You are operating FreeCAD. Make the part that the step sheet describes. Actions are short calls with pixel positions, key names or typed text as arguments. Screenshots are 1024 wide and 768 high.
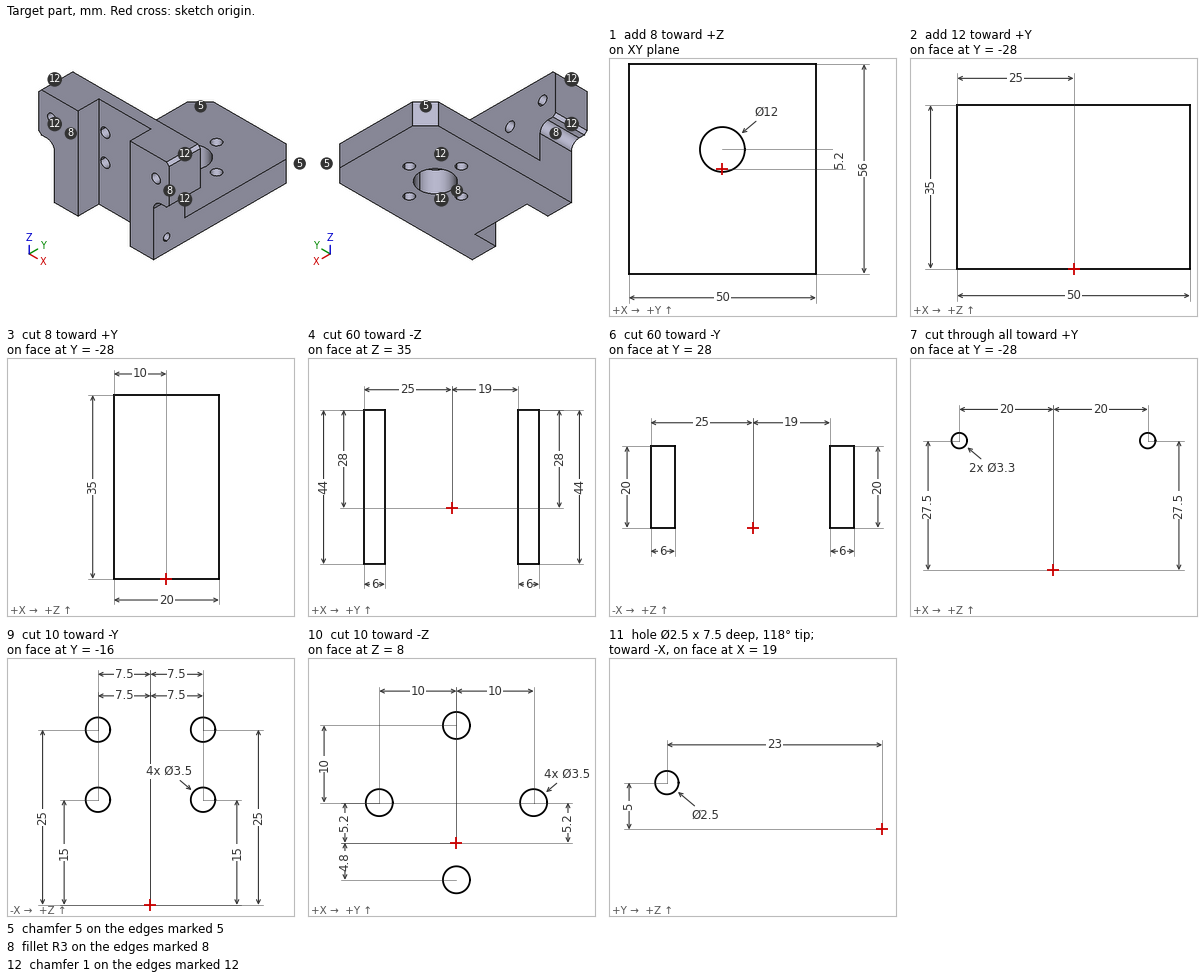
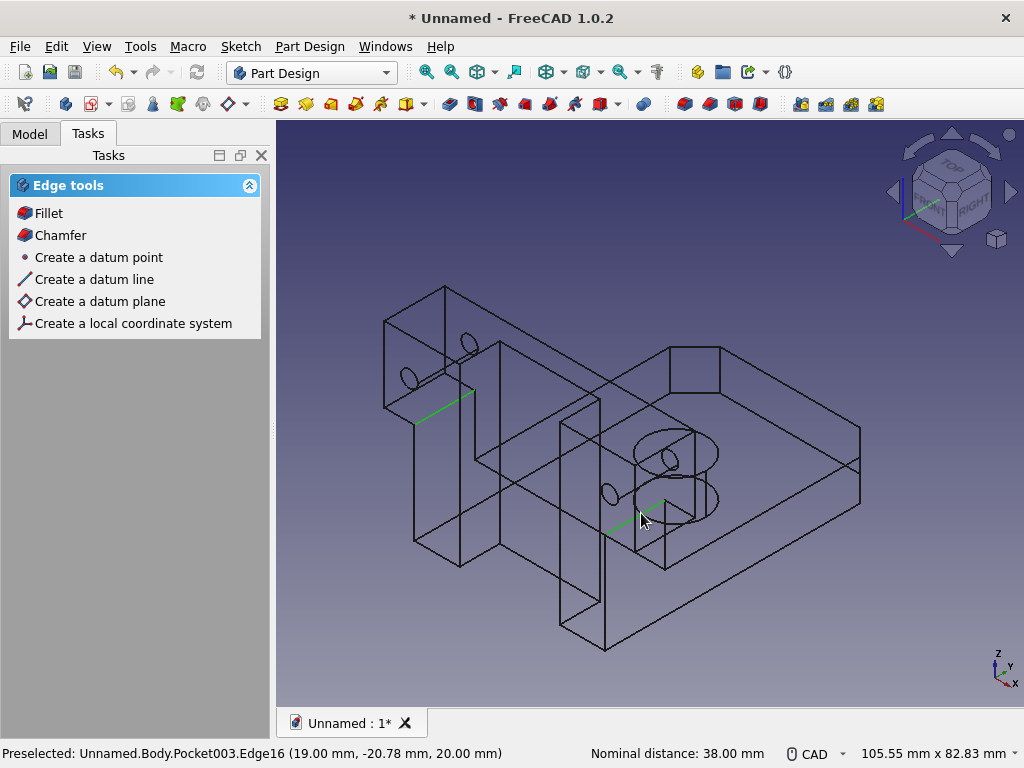
key(v)
key(1)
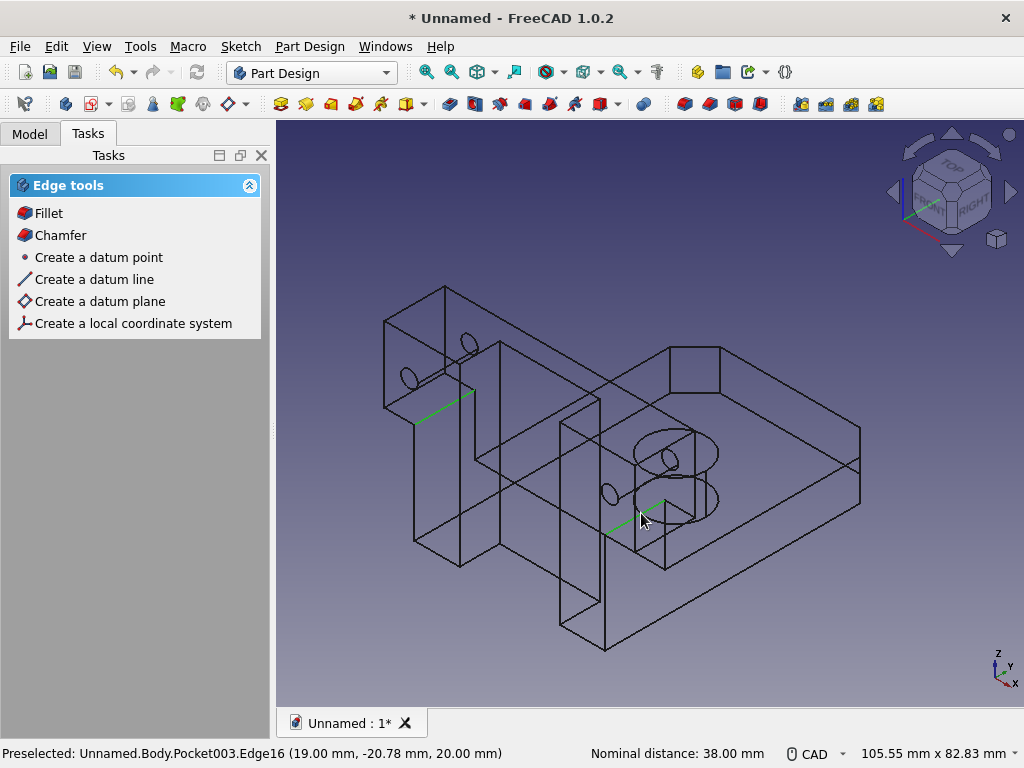
click(685, 104)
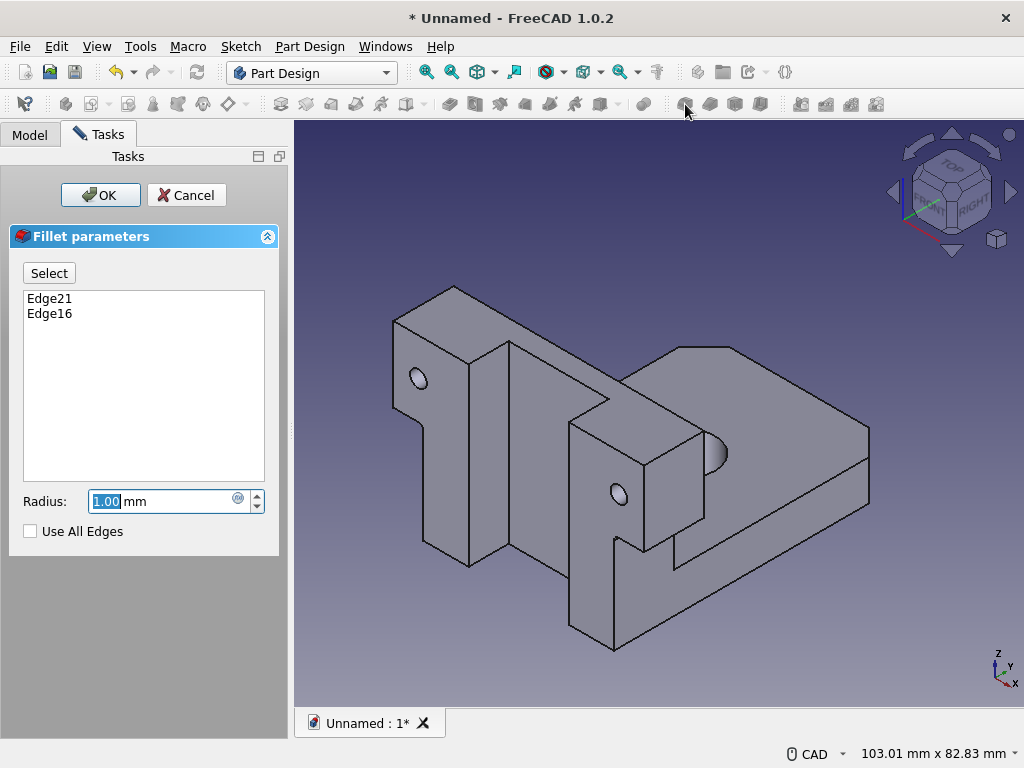
text(3)
key(Tab)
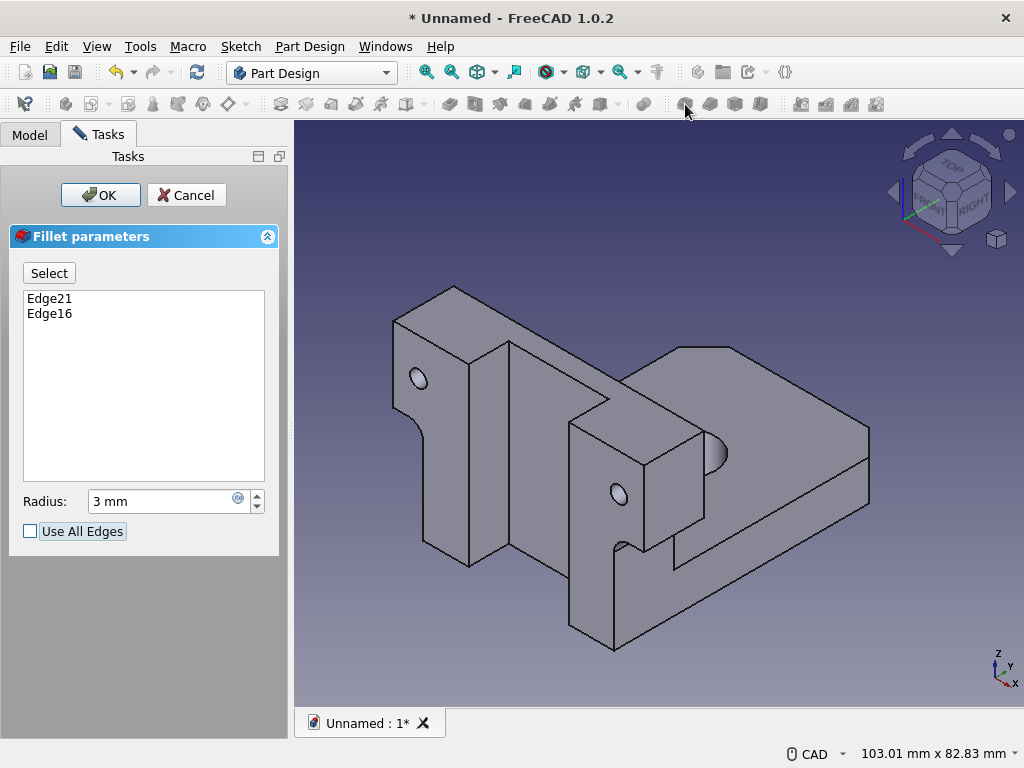
click(101, 195)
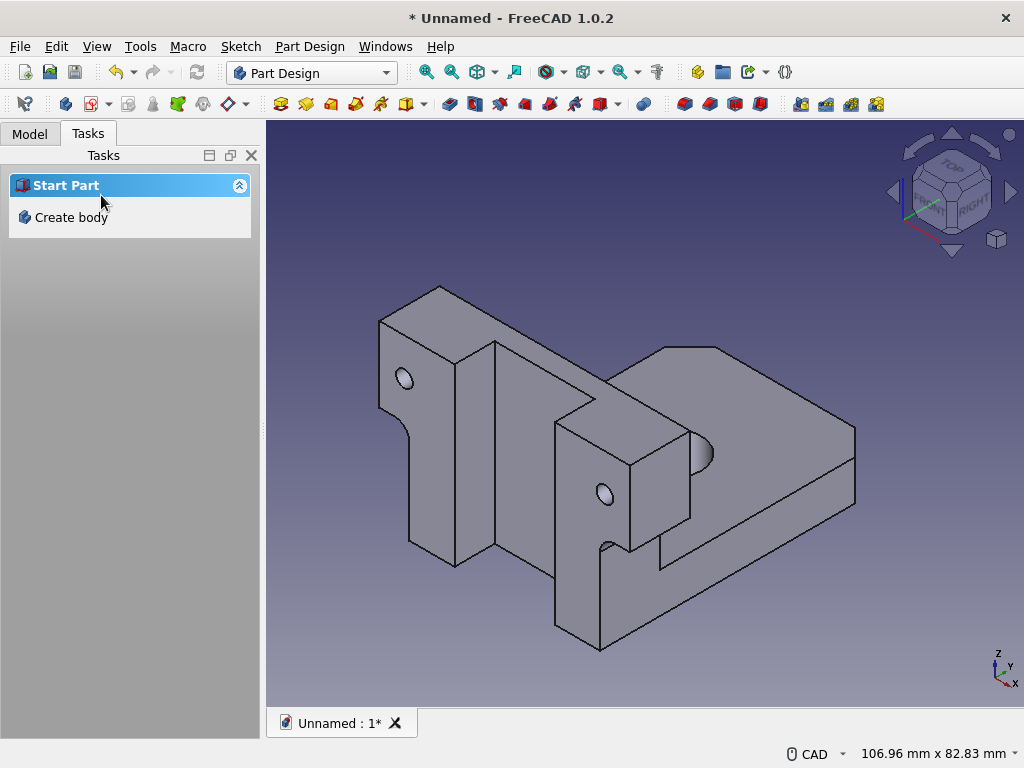
key(4)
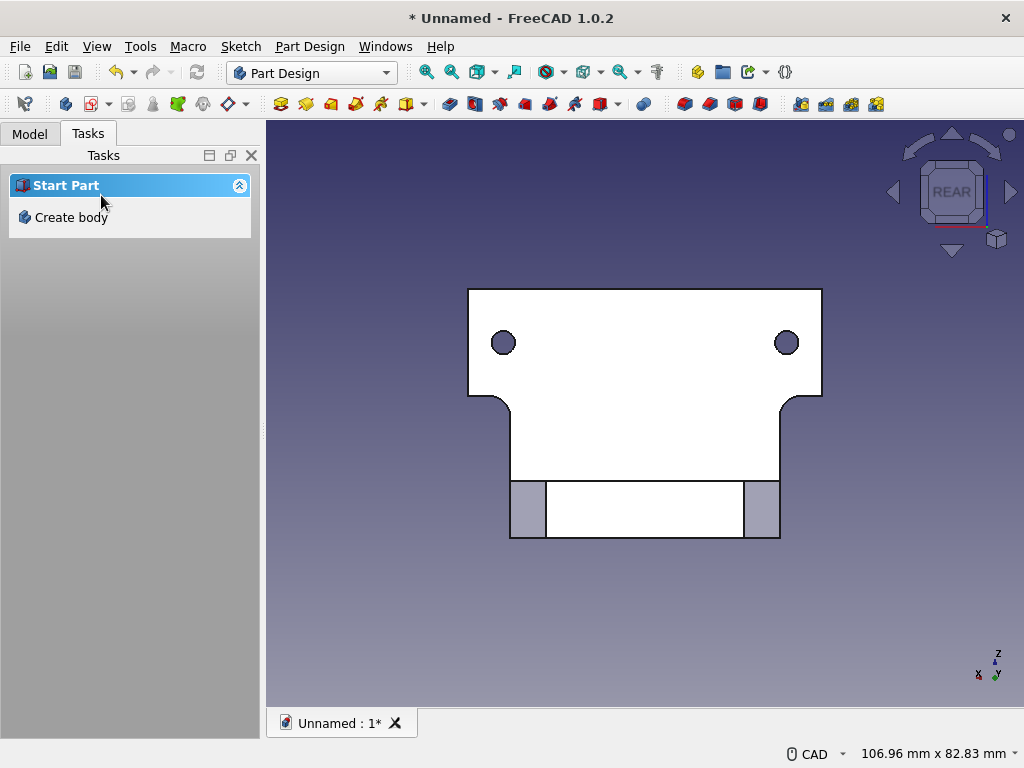
click(645, 384)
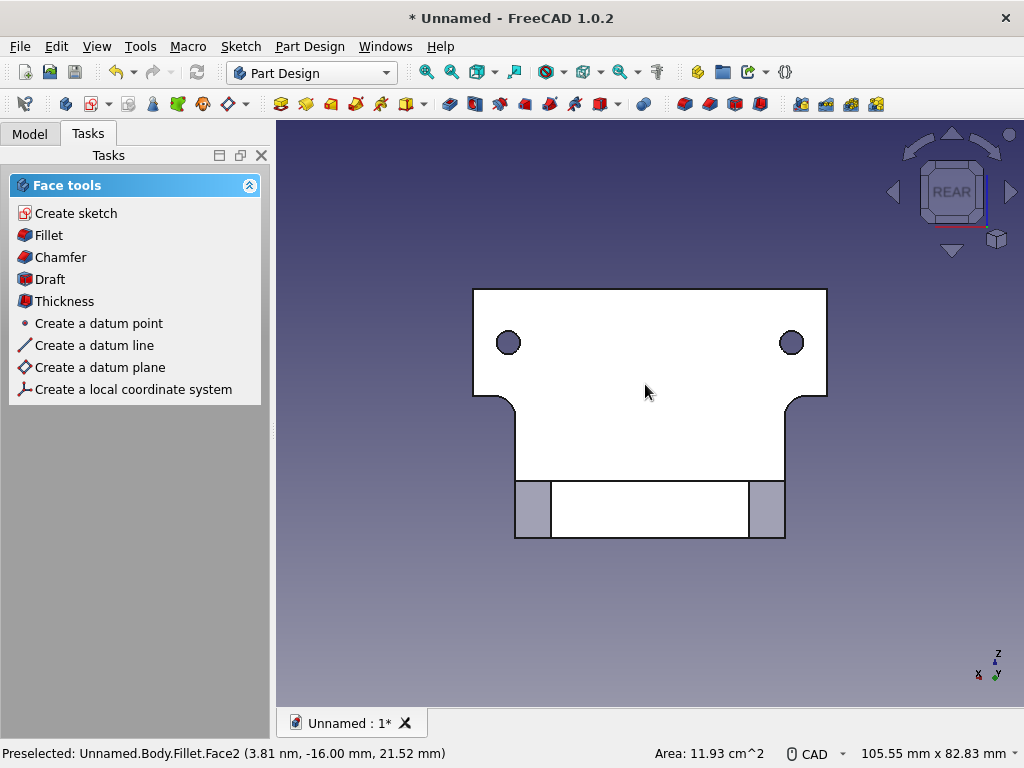
click(90, 104)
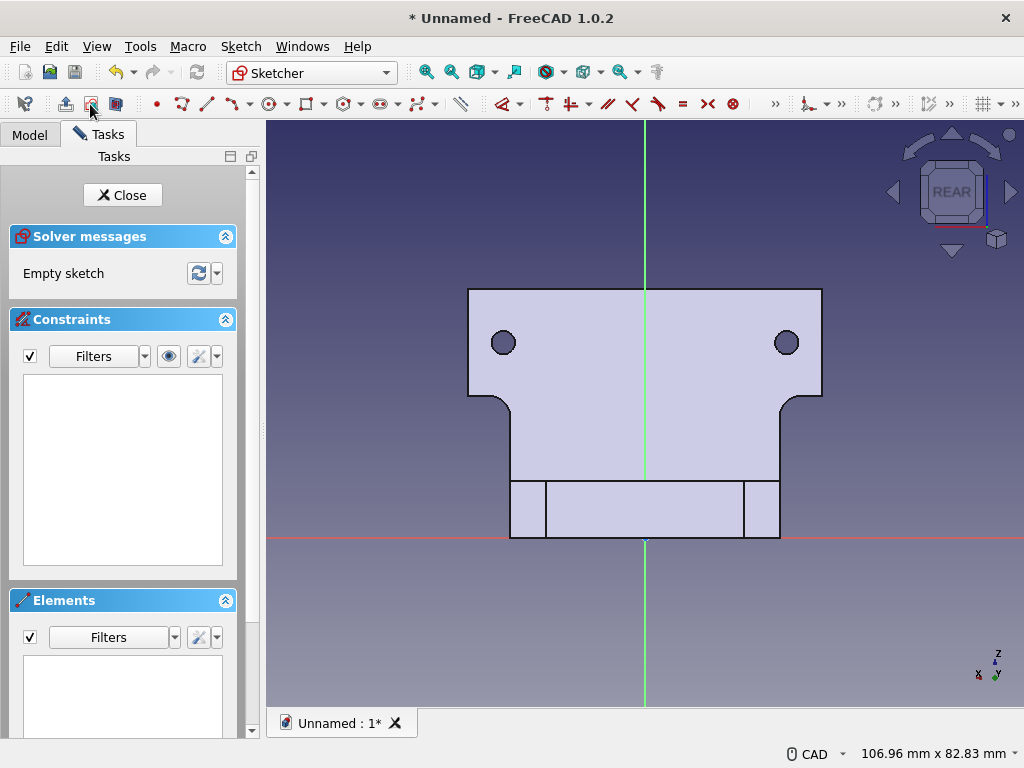
click(116, 104)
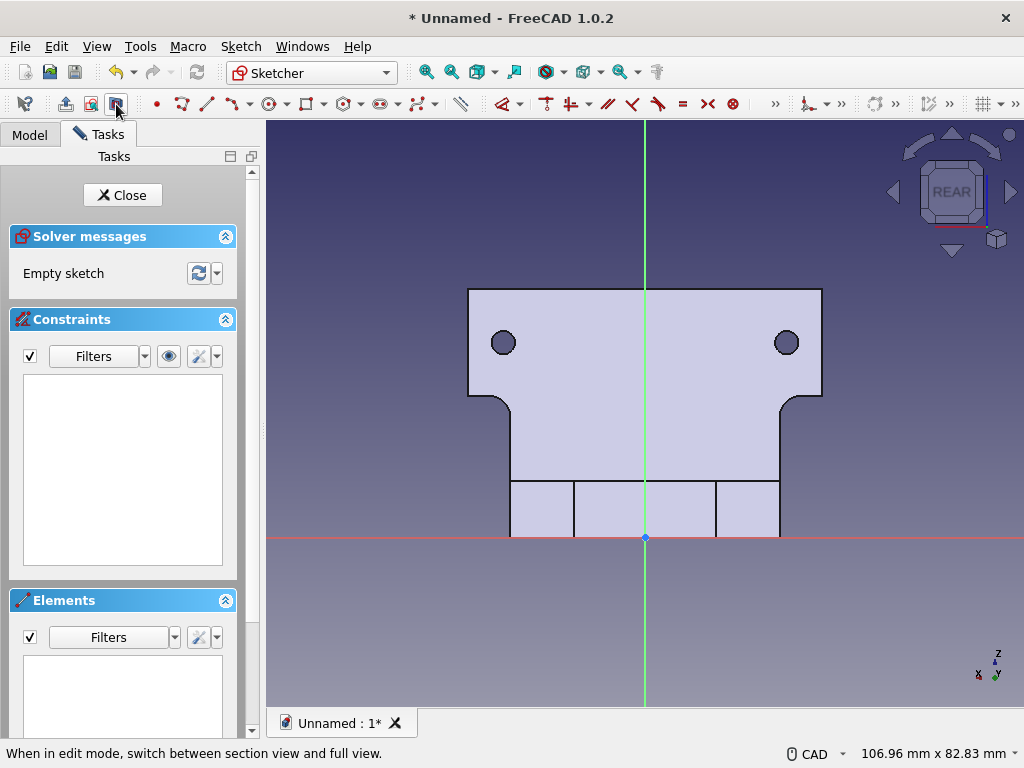
scroll(728, 478, up, 3)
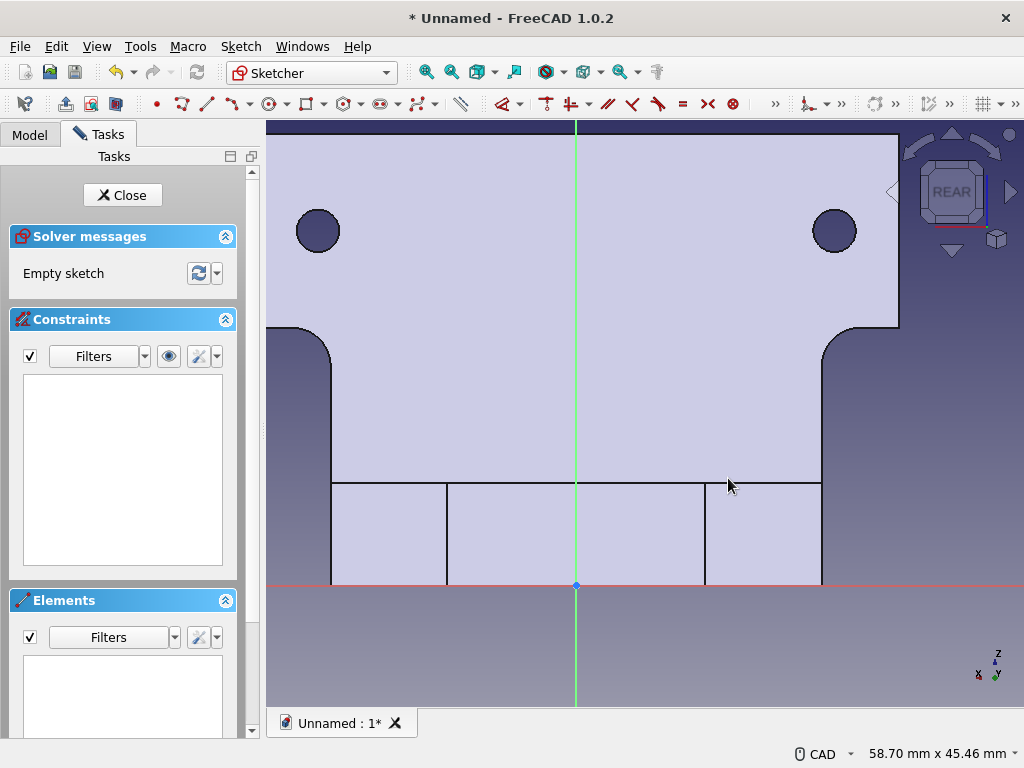
click(268, 104)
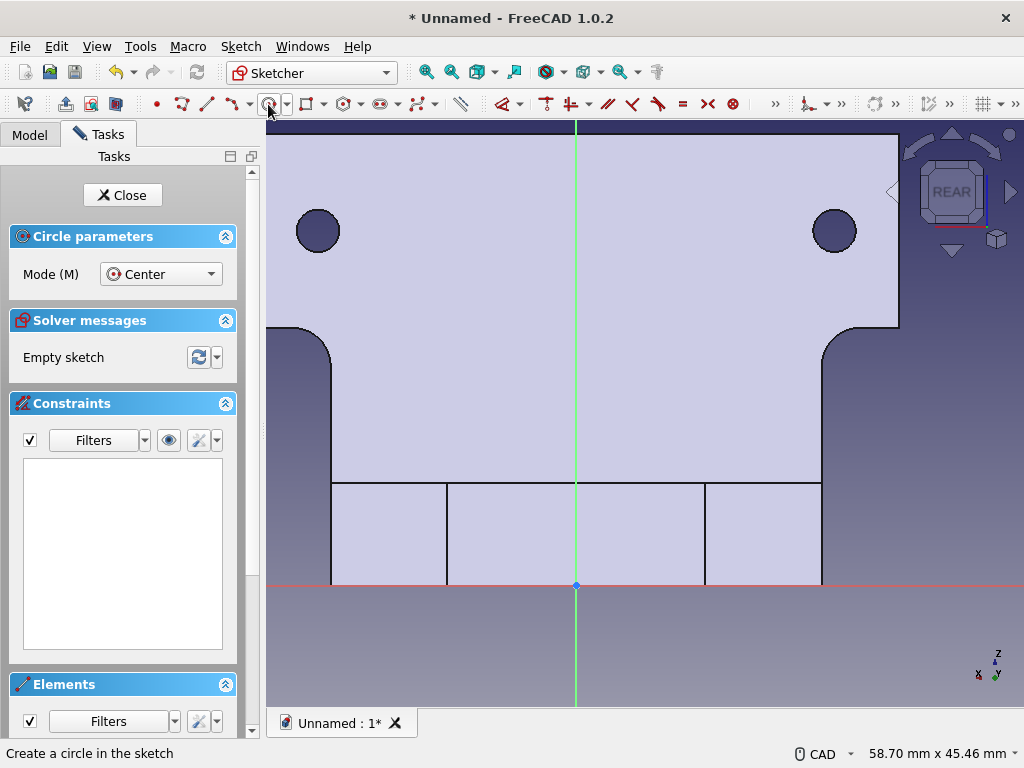
click(673, 392)
move(689, 376)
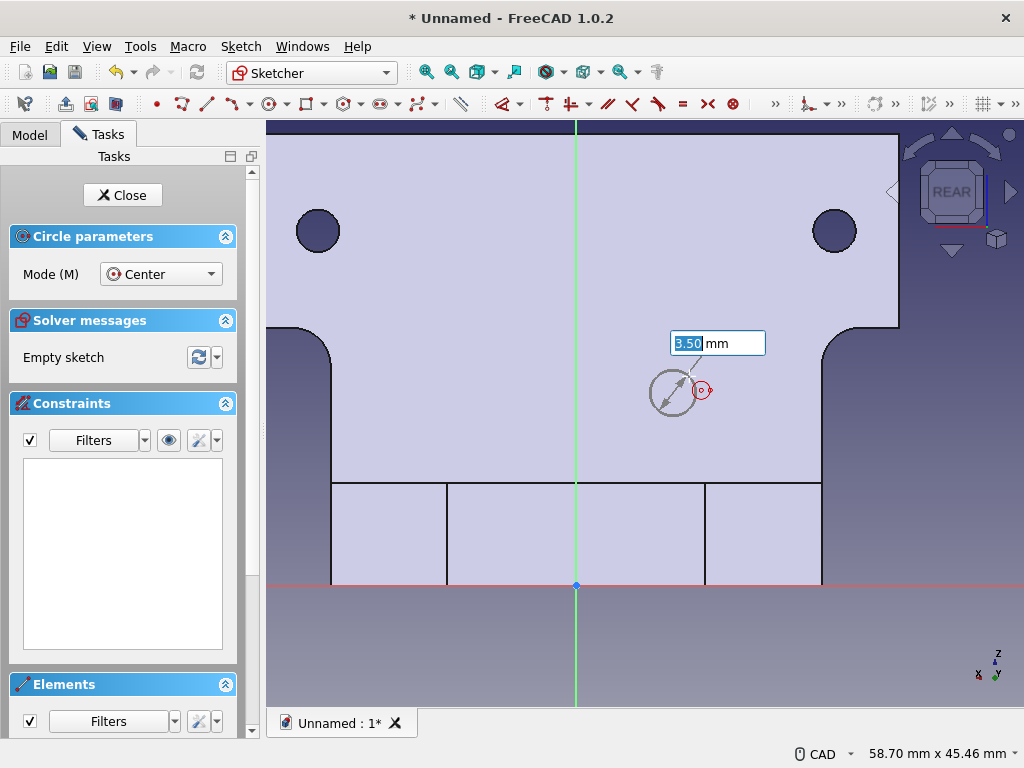
text(3.5)
key(Return)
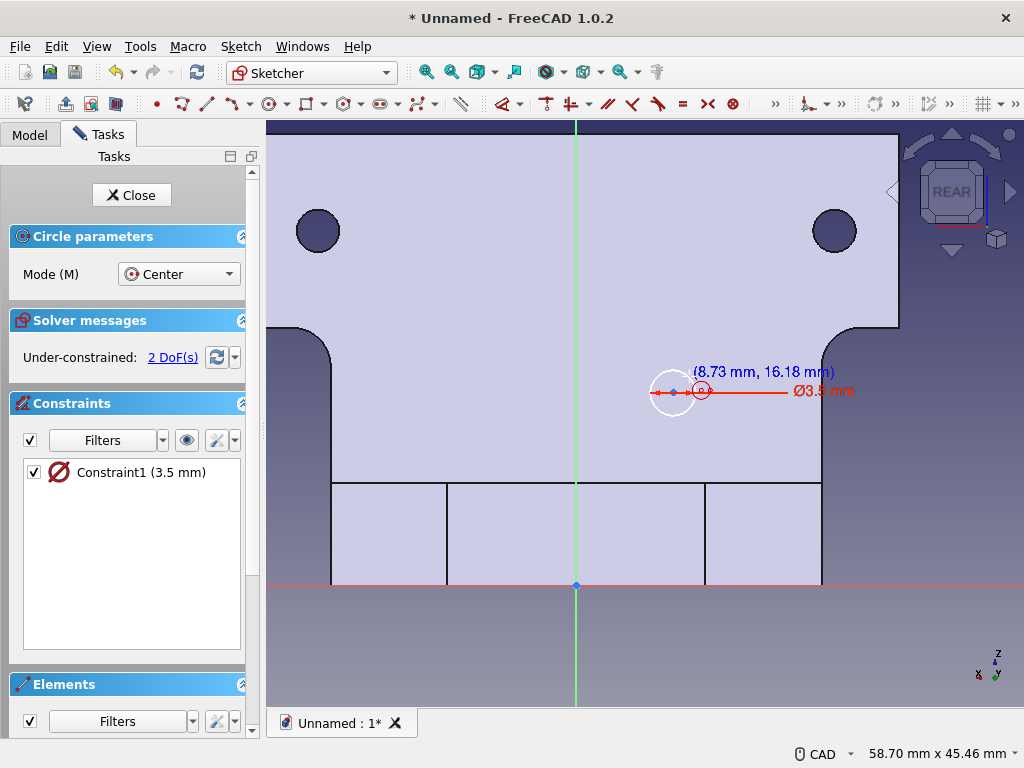
click(479, 392)
move(495, 376)